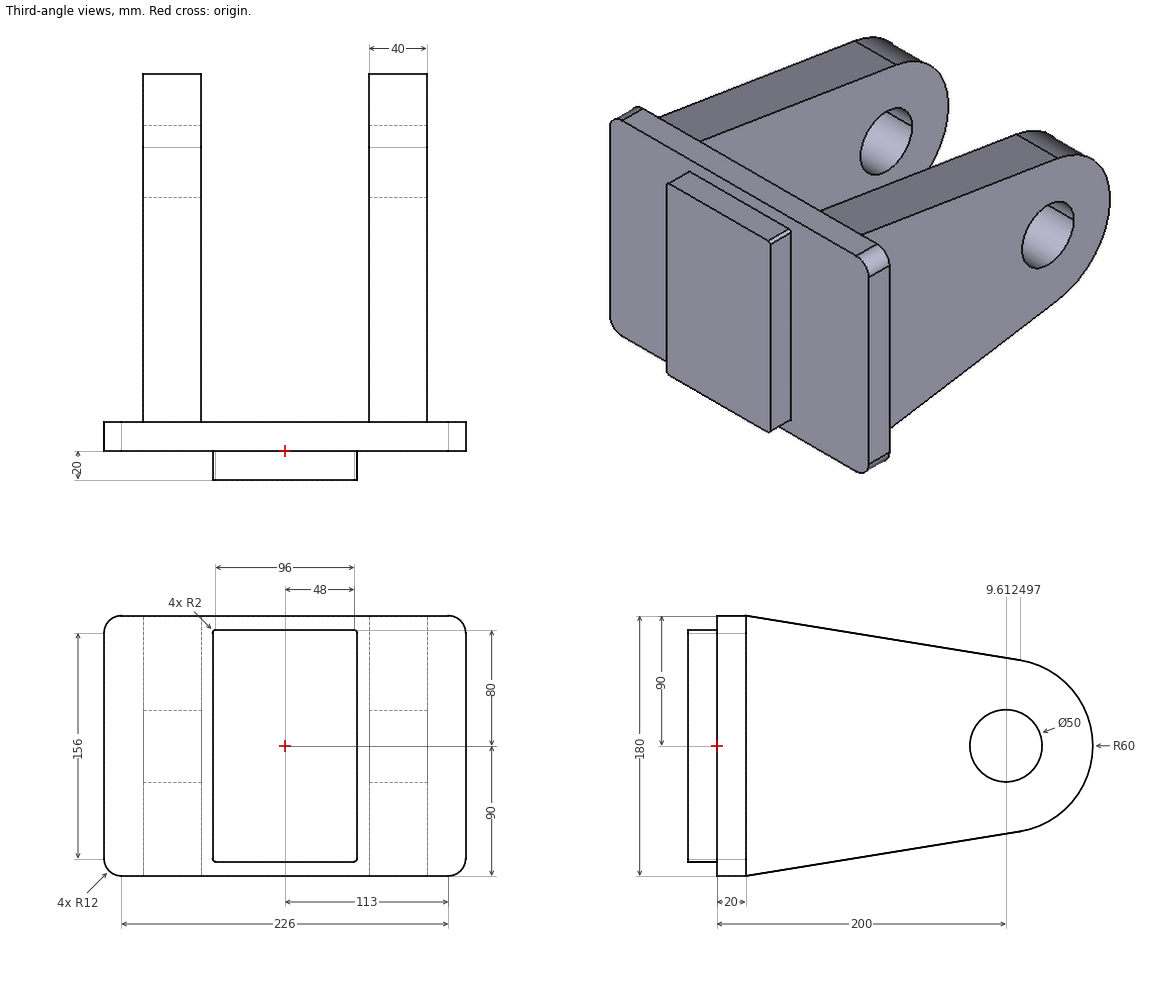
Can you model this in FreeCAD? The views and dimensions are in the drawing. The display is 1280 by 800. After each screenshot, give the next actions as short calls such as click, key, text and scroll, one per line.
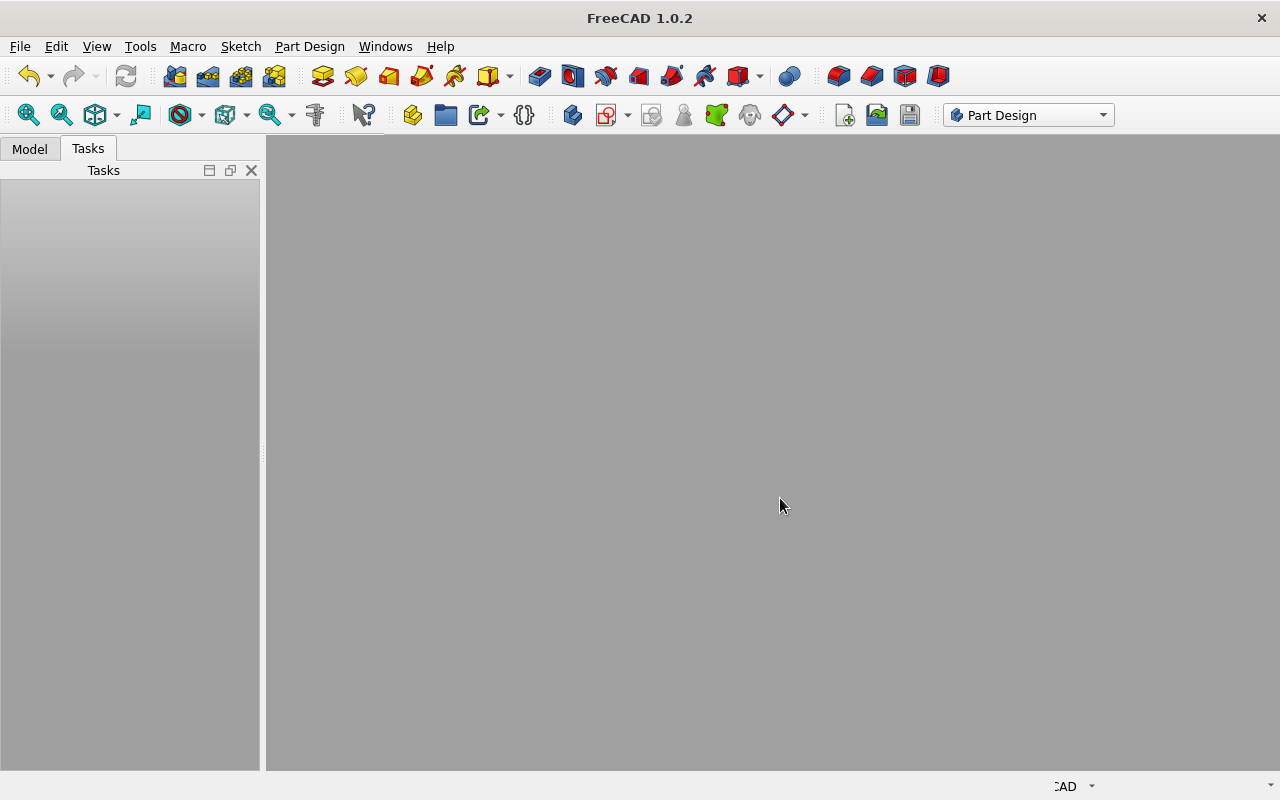
click(844, 116)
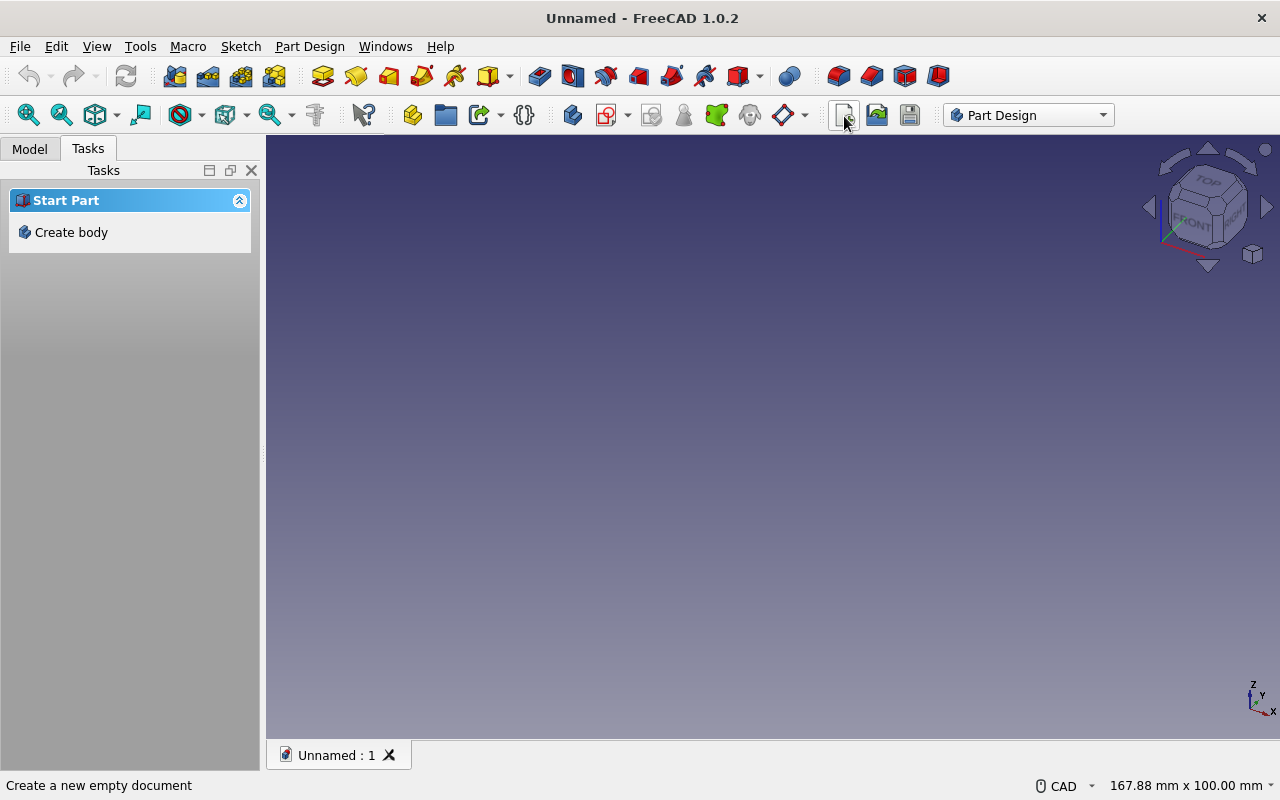
click(606, 116)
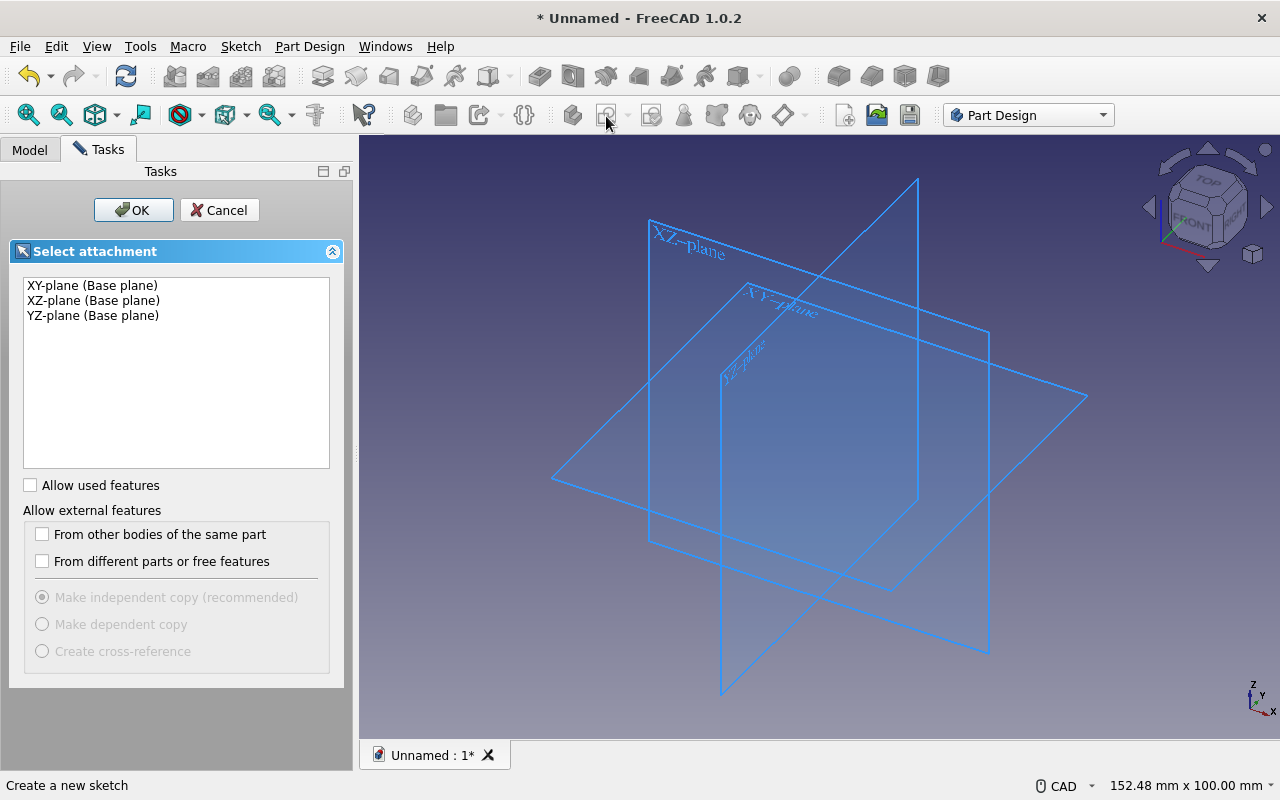
click(84, 300)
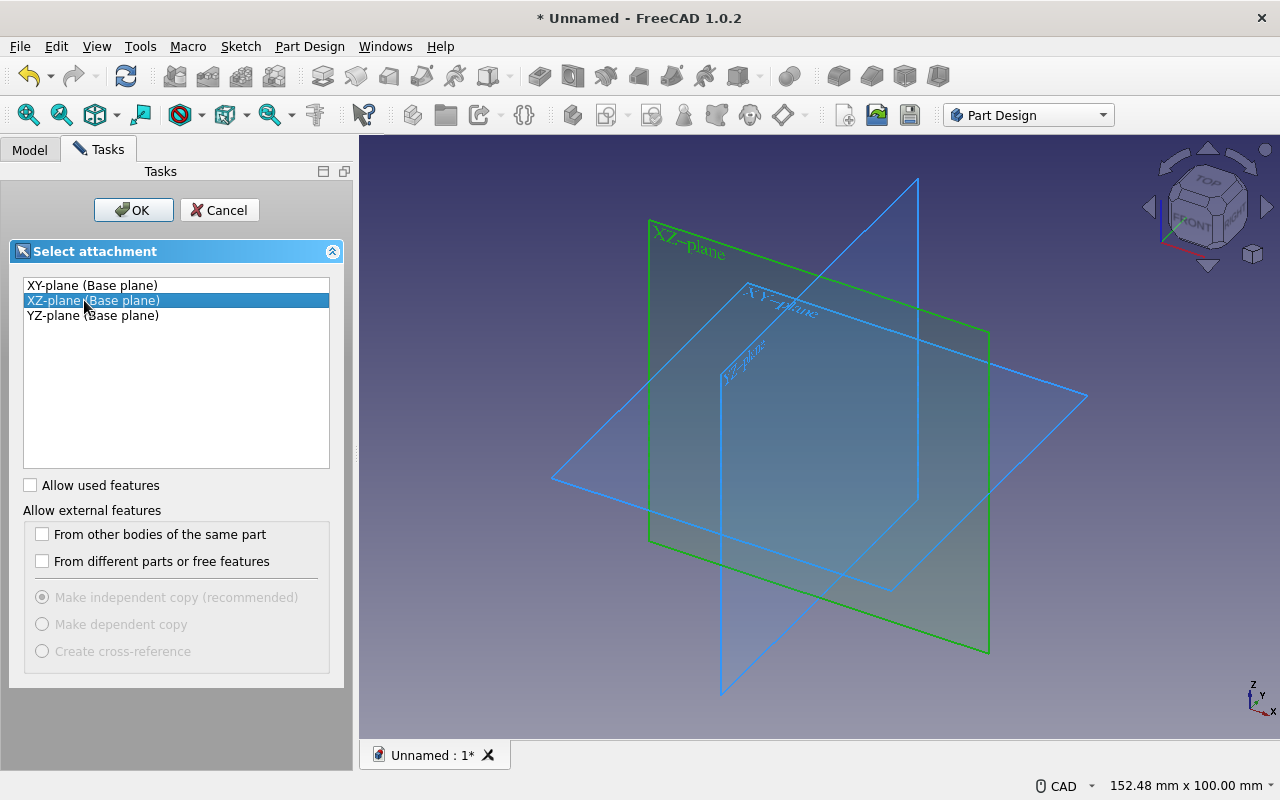
click(134, 210)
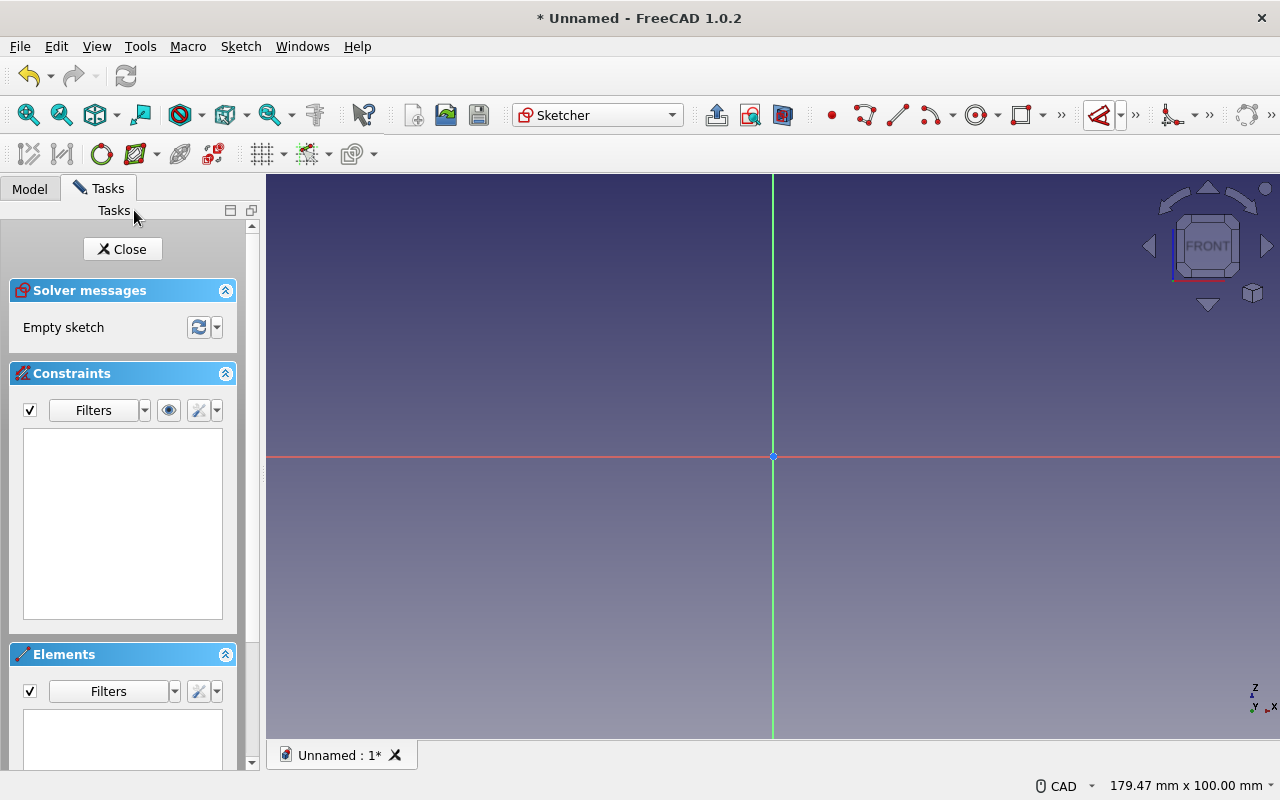
scroll(665, 456, down, 5)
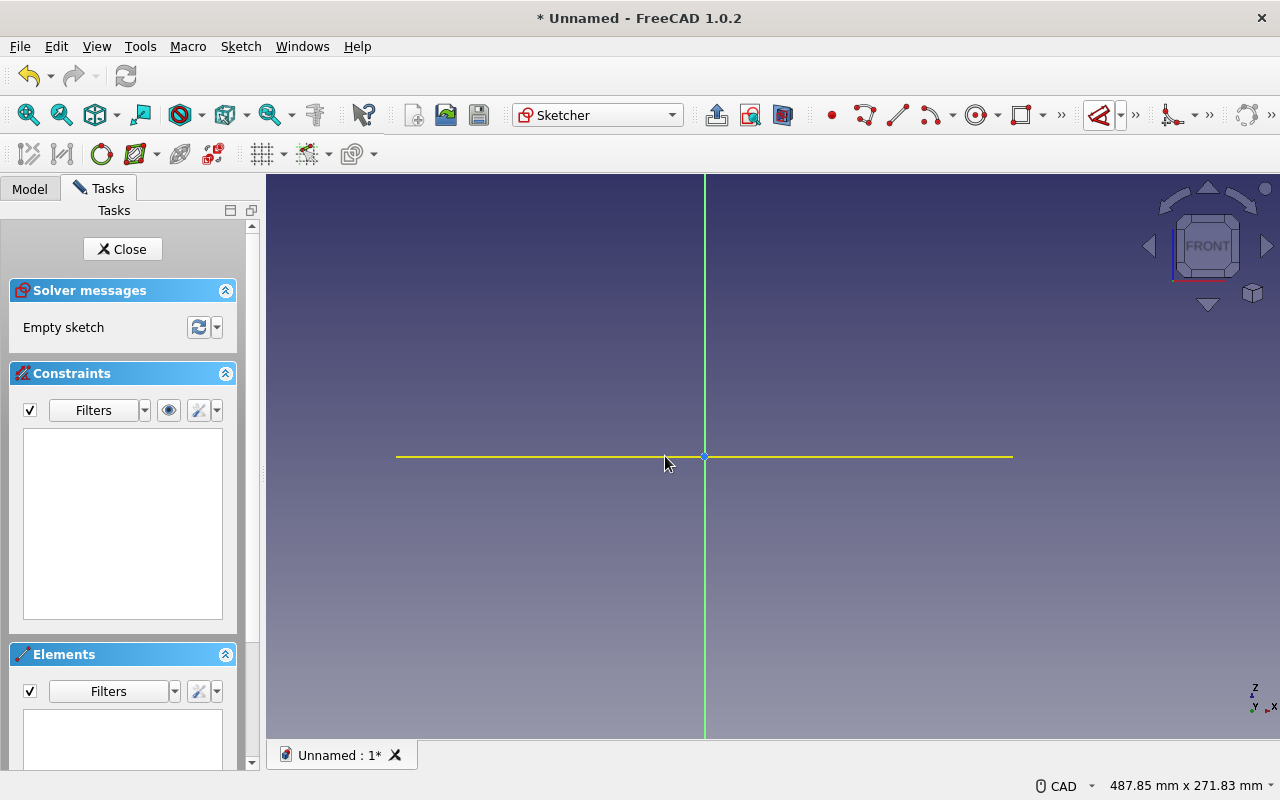
click(898, 116)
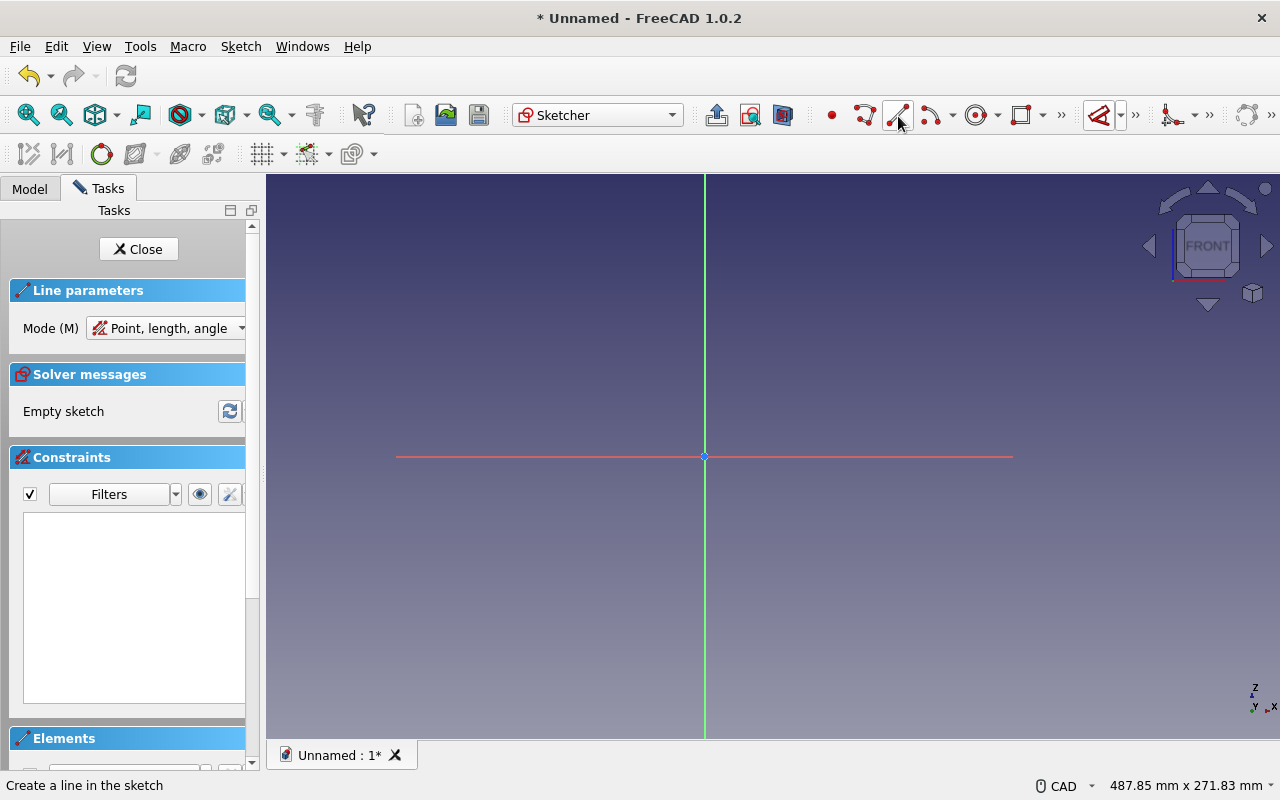
click(940, 644)
click(470, 644)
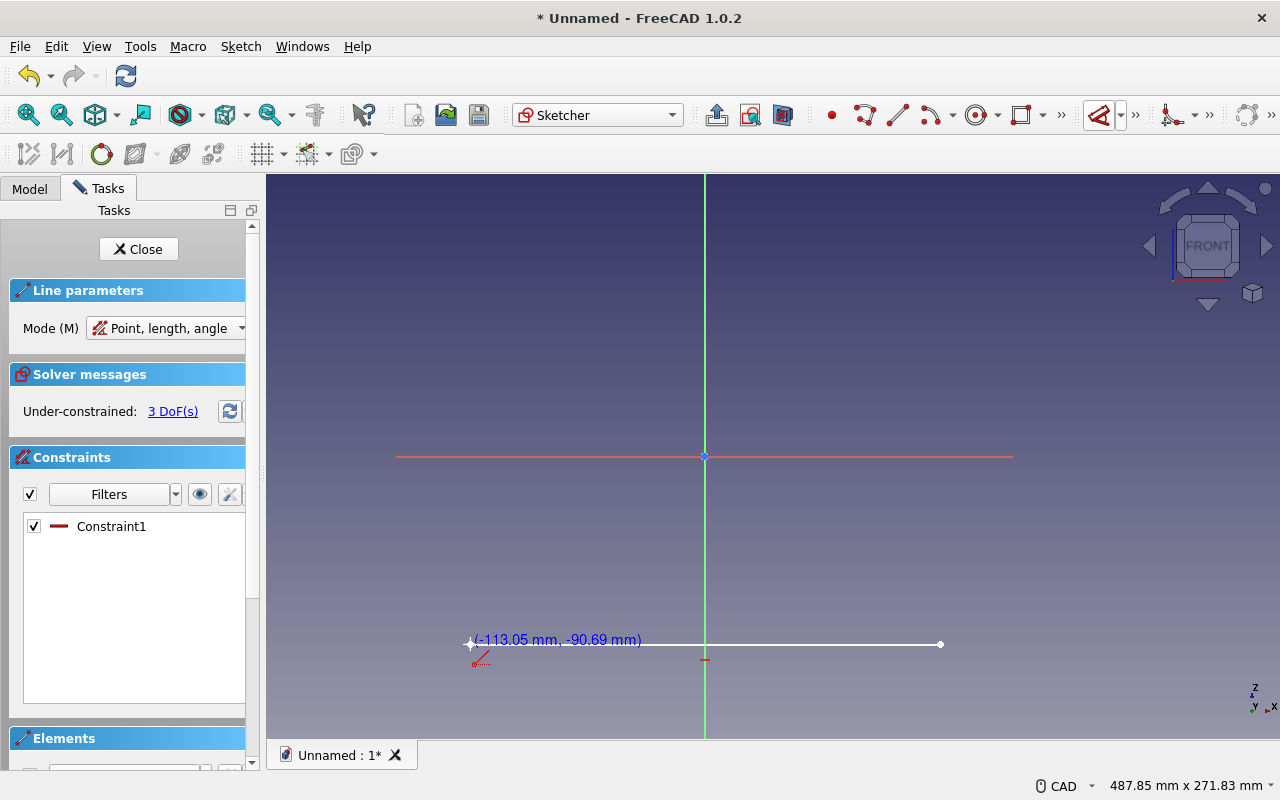
click(445, 619)
click(445, 294)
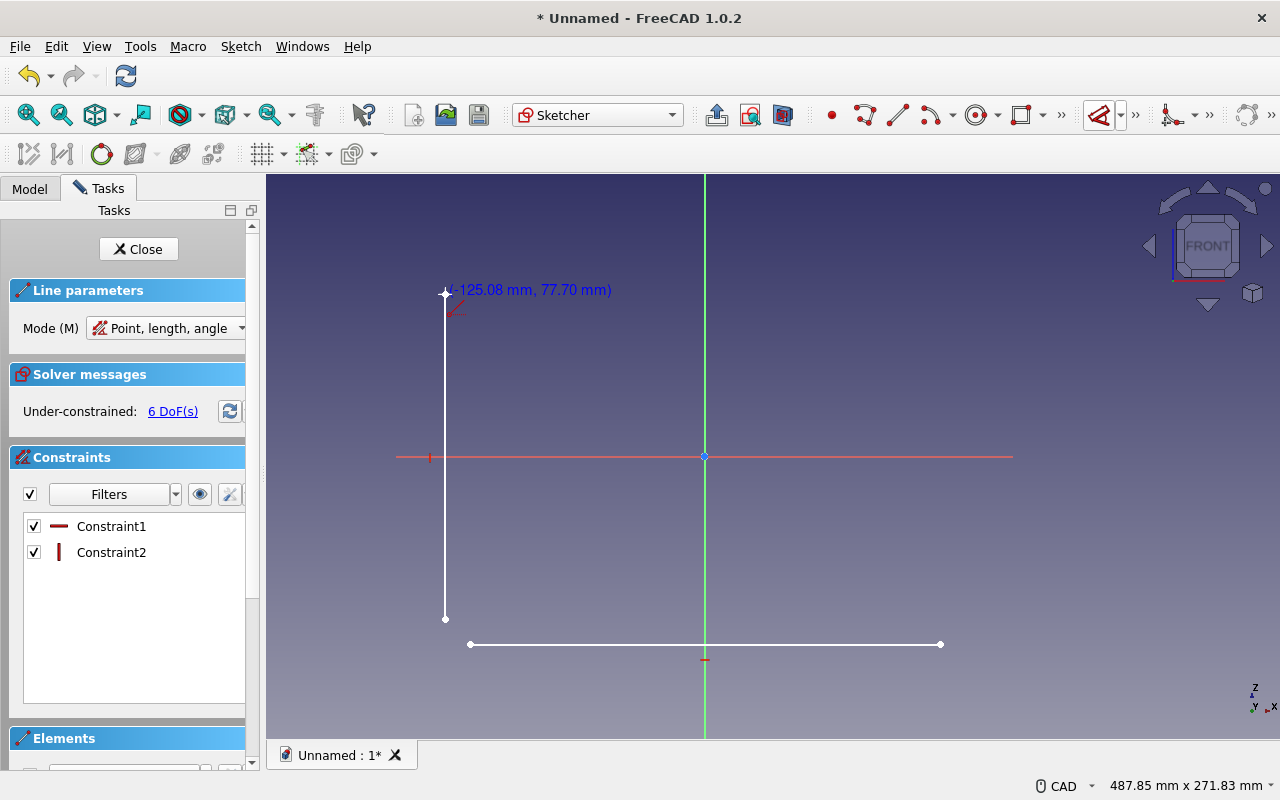
click(470, 269)
click(940, 269)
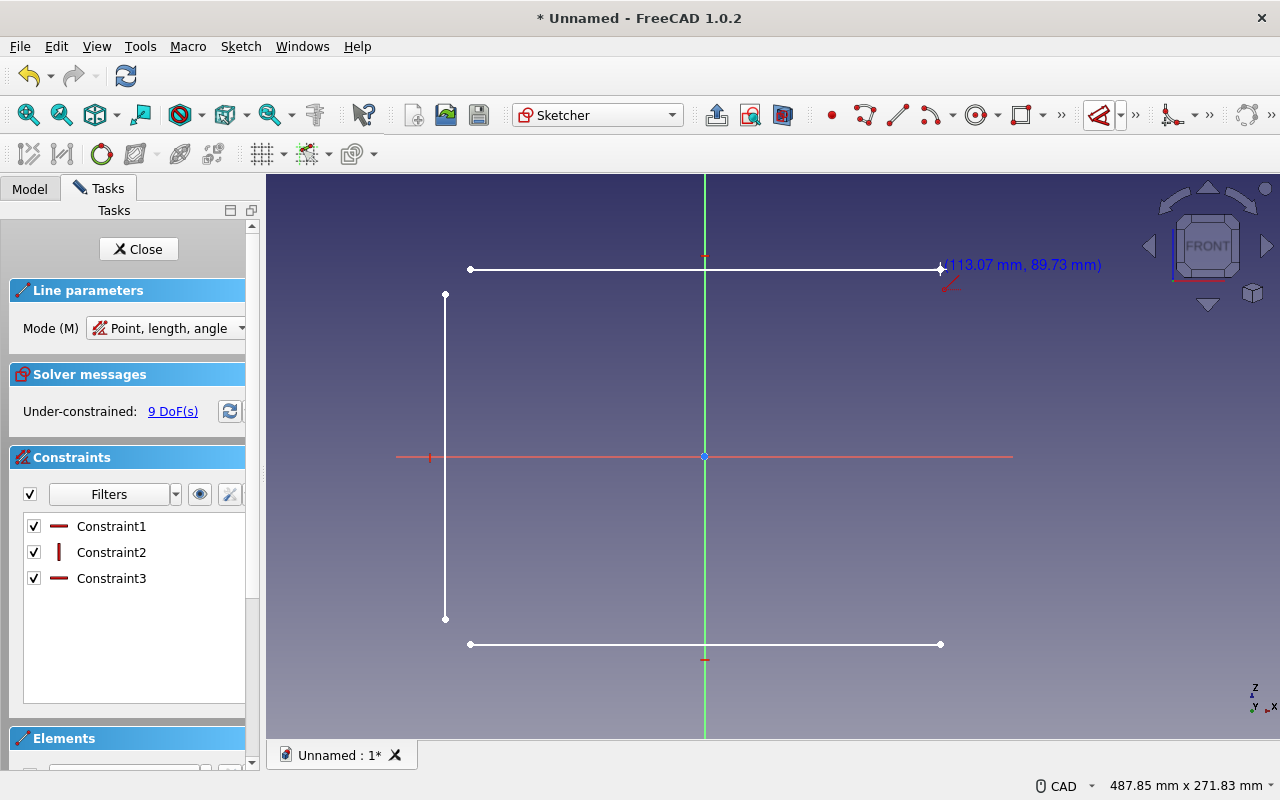
click(965, 294)
click(965, 619)